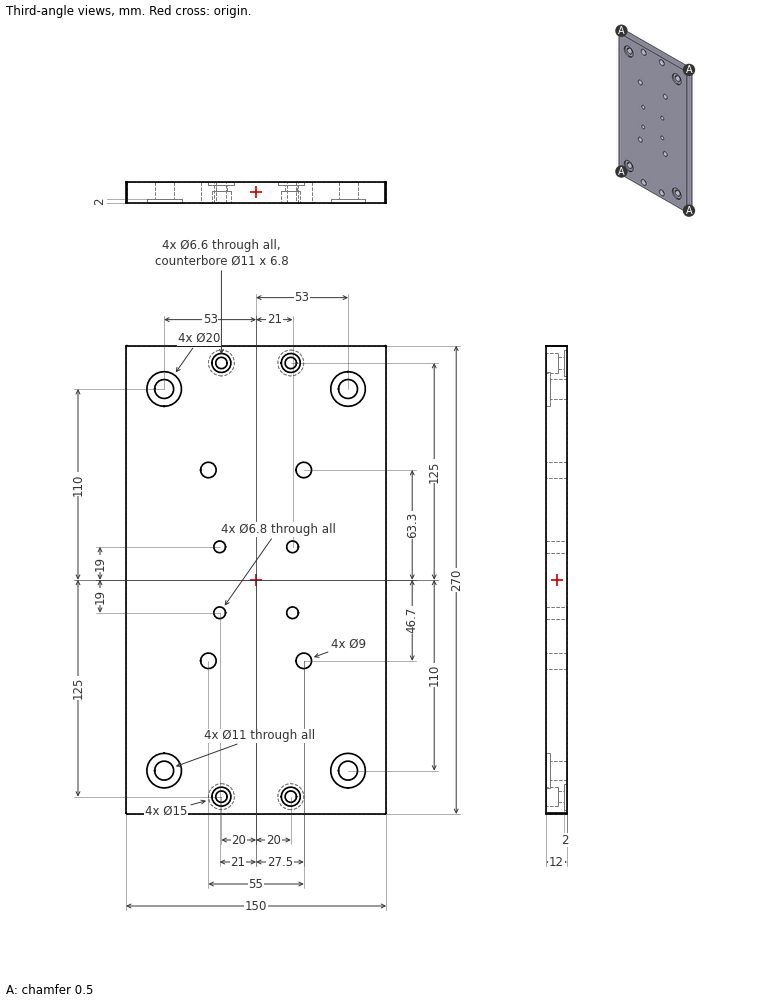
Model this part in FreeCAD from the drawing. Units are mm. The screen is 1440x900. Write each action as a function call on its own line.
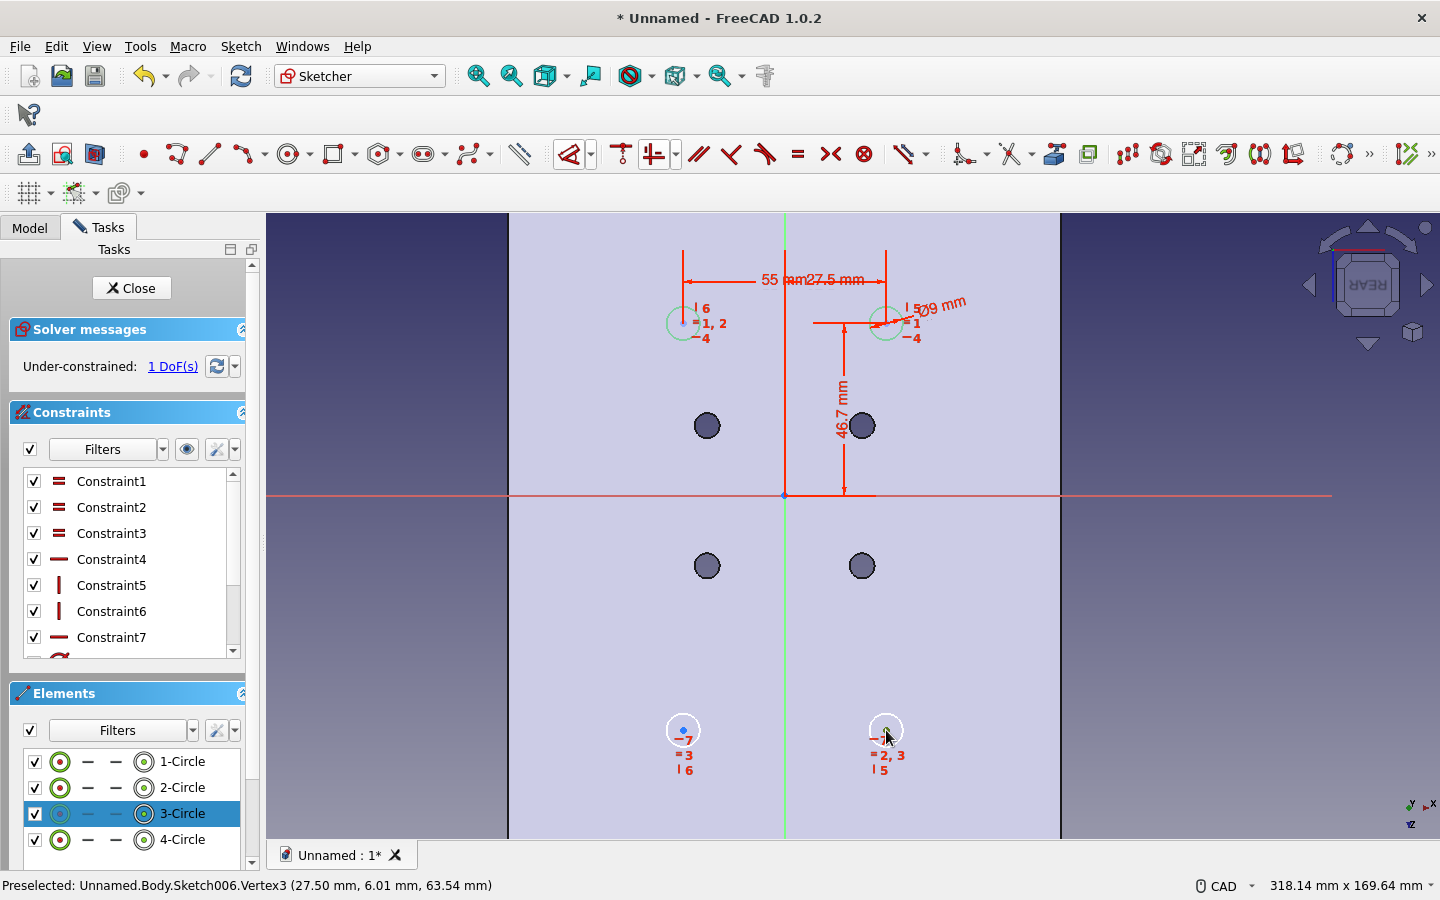
key(i)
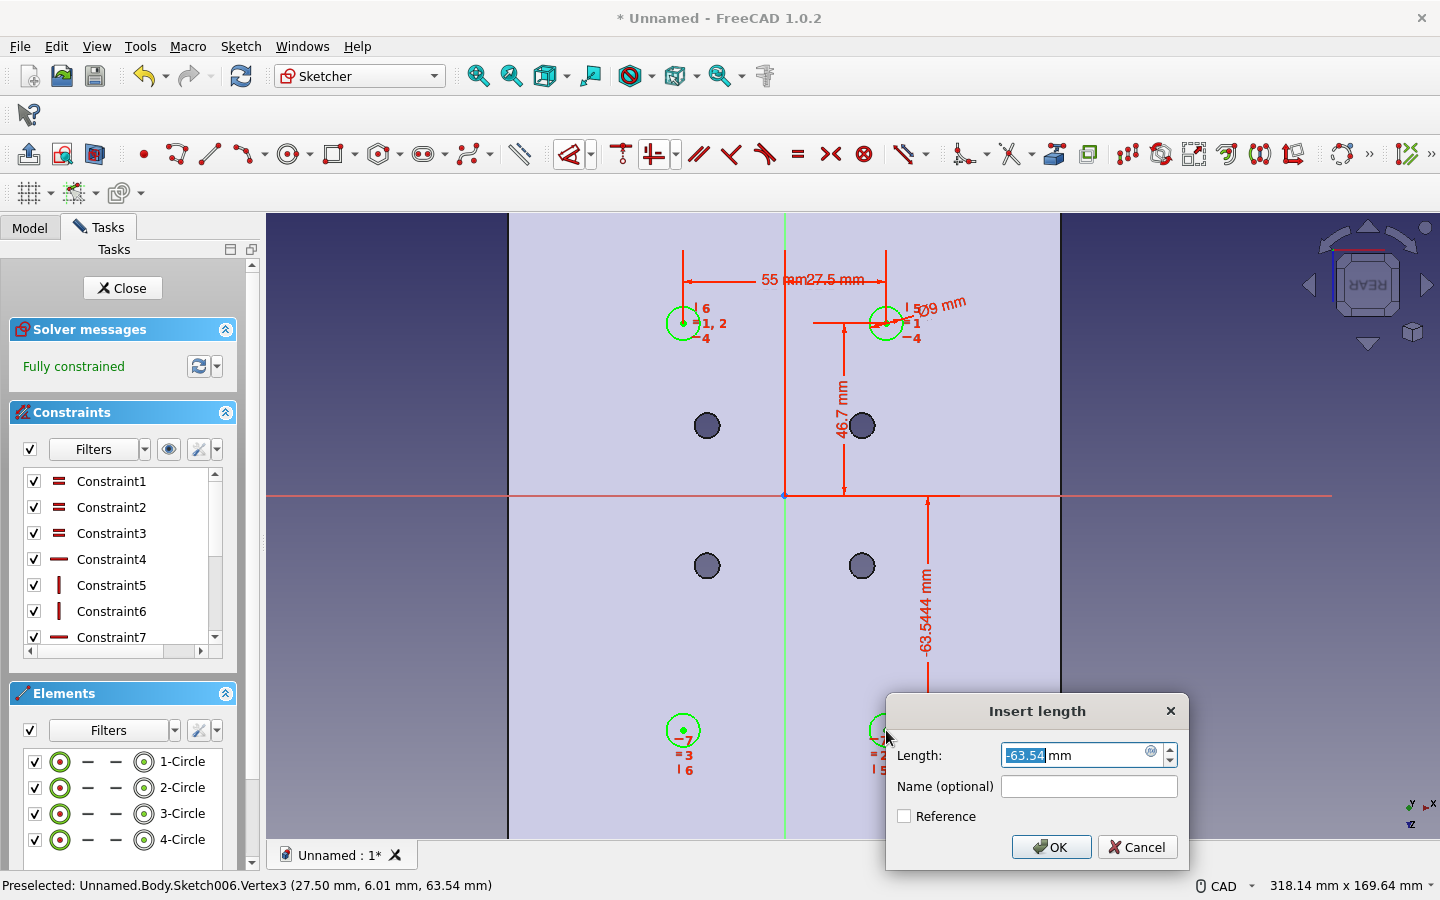
text(-63.3)
key(Return)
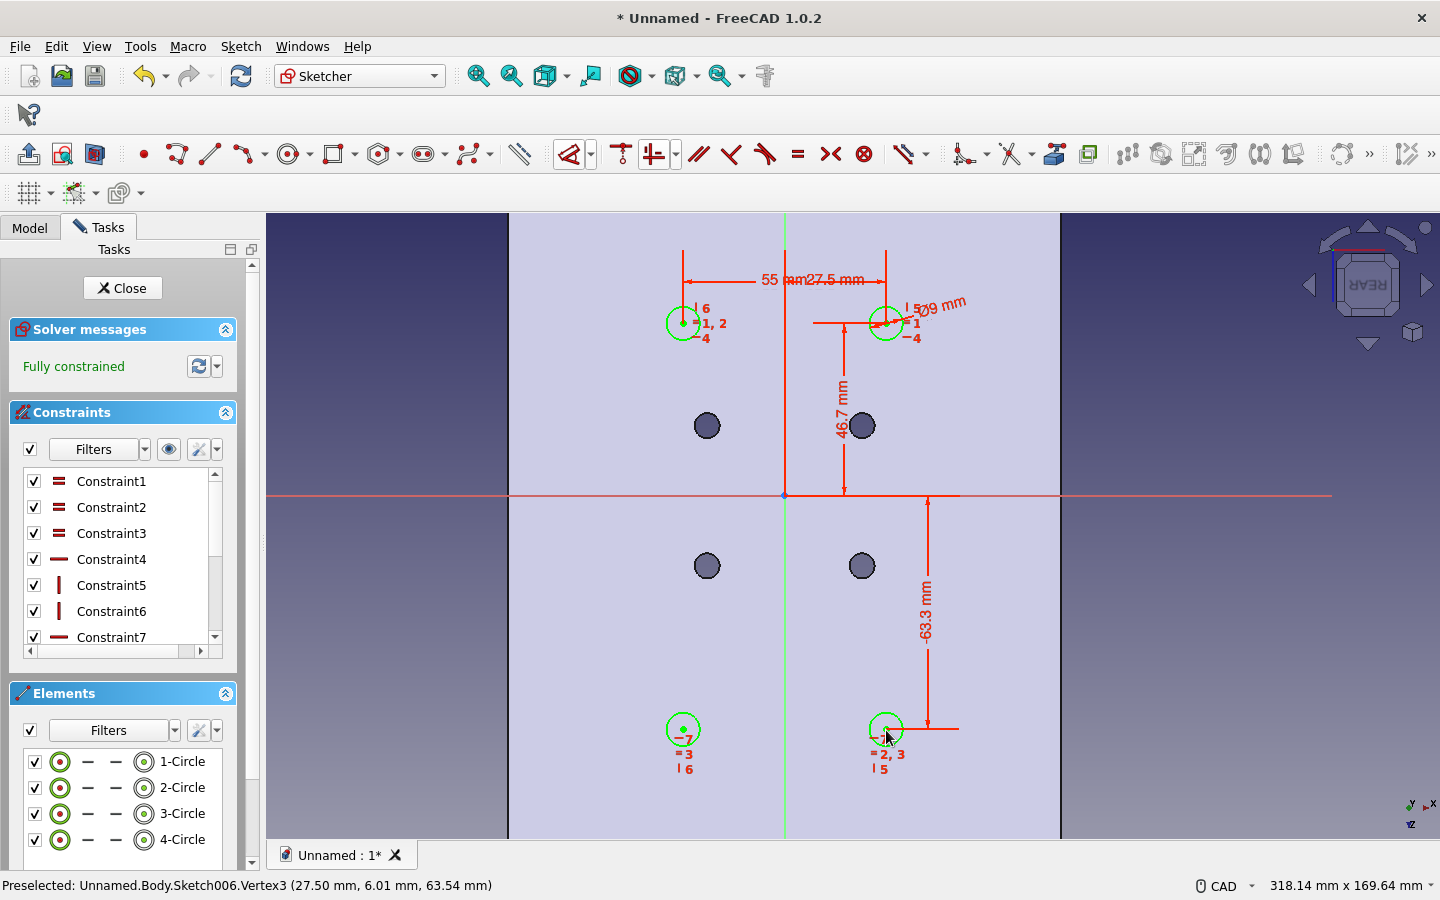
click(123, 288)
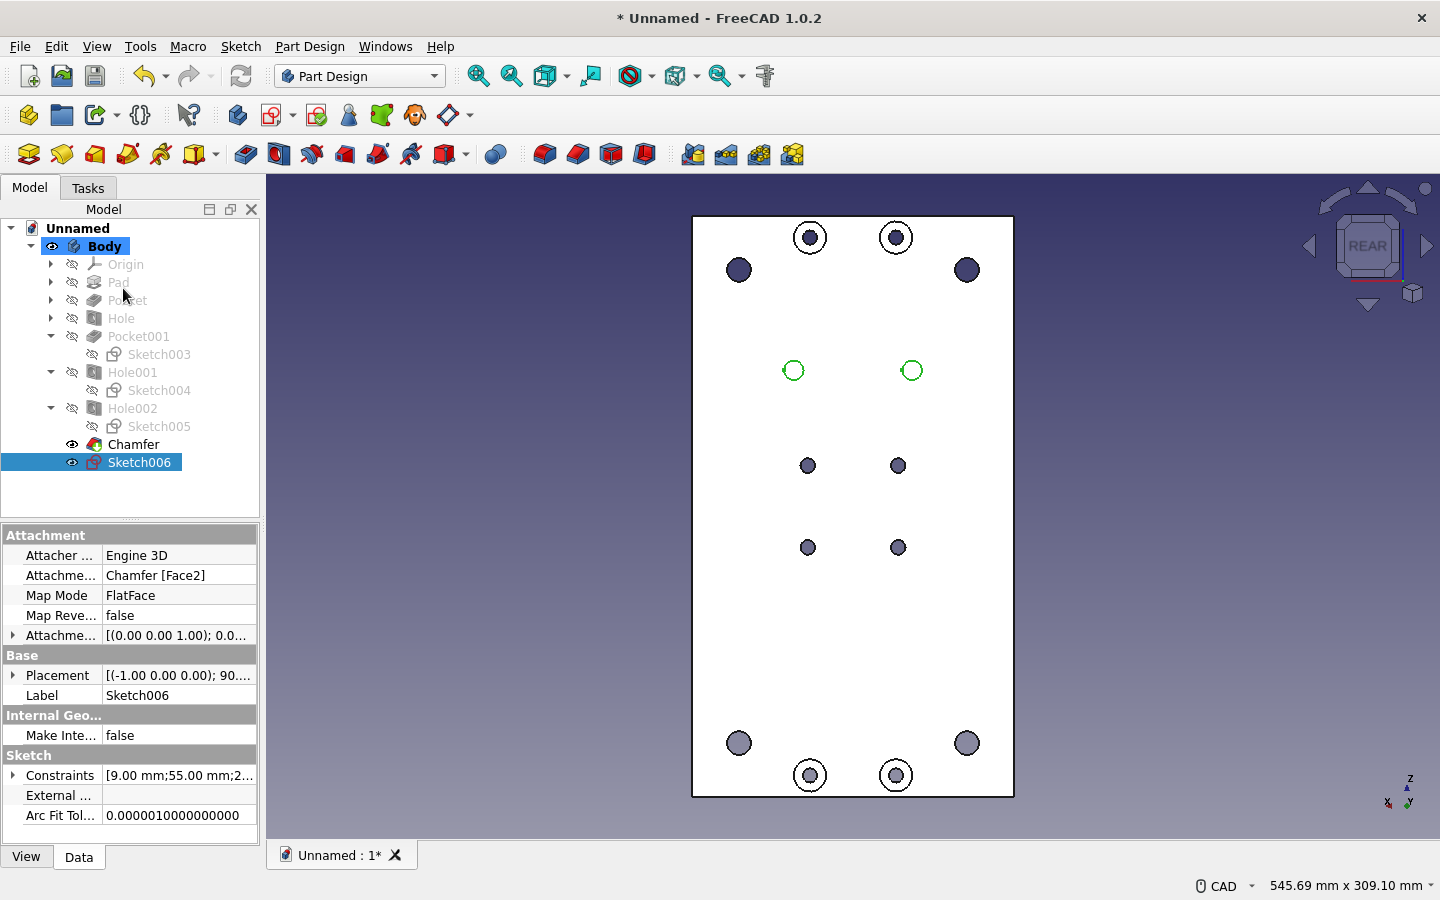
click(246, 154)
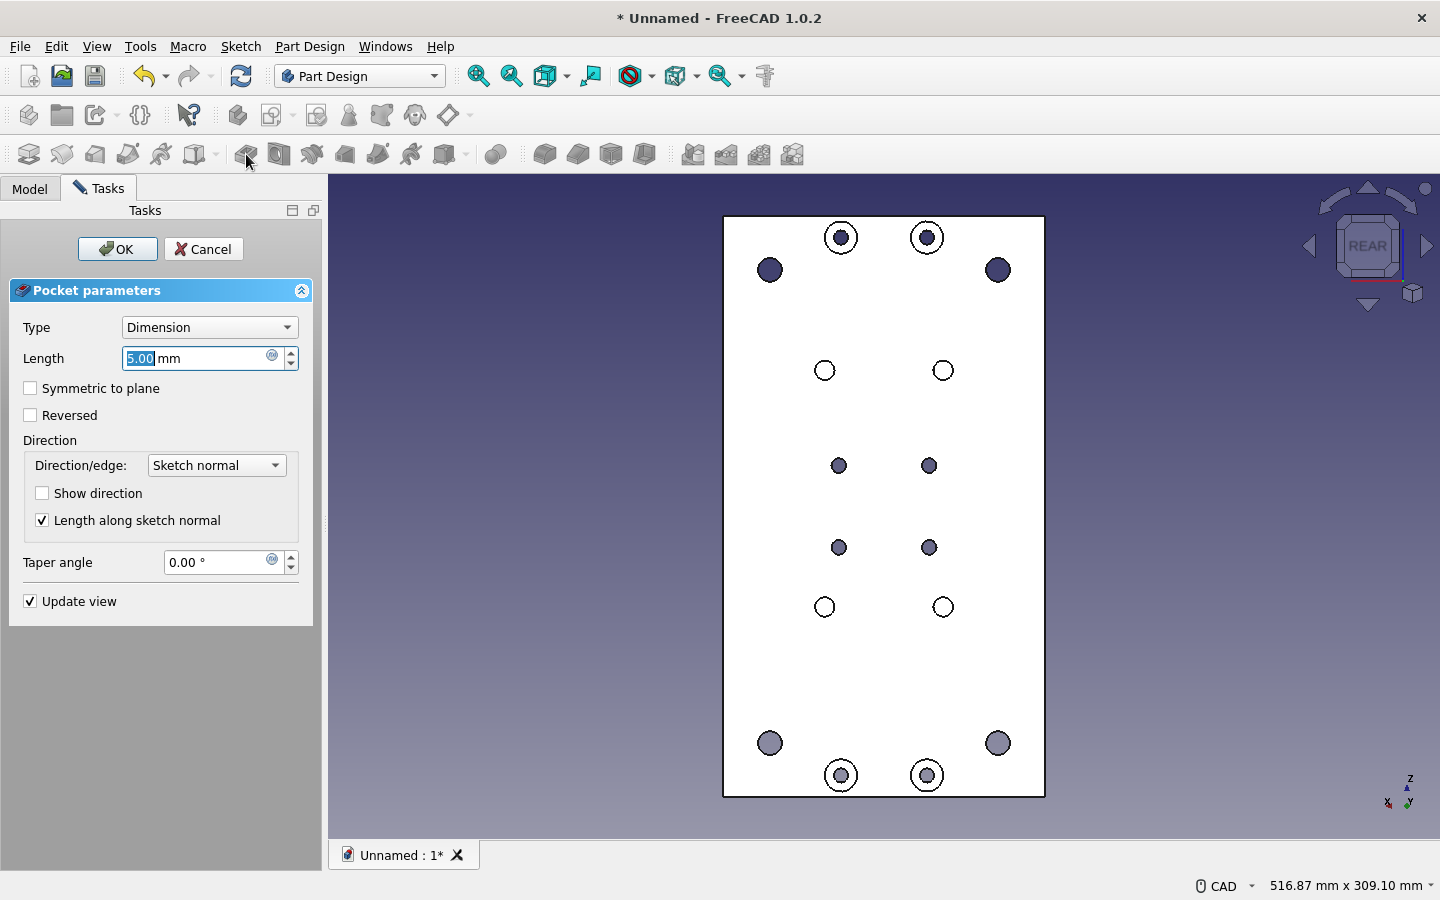
click(210, 328)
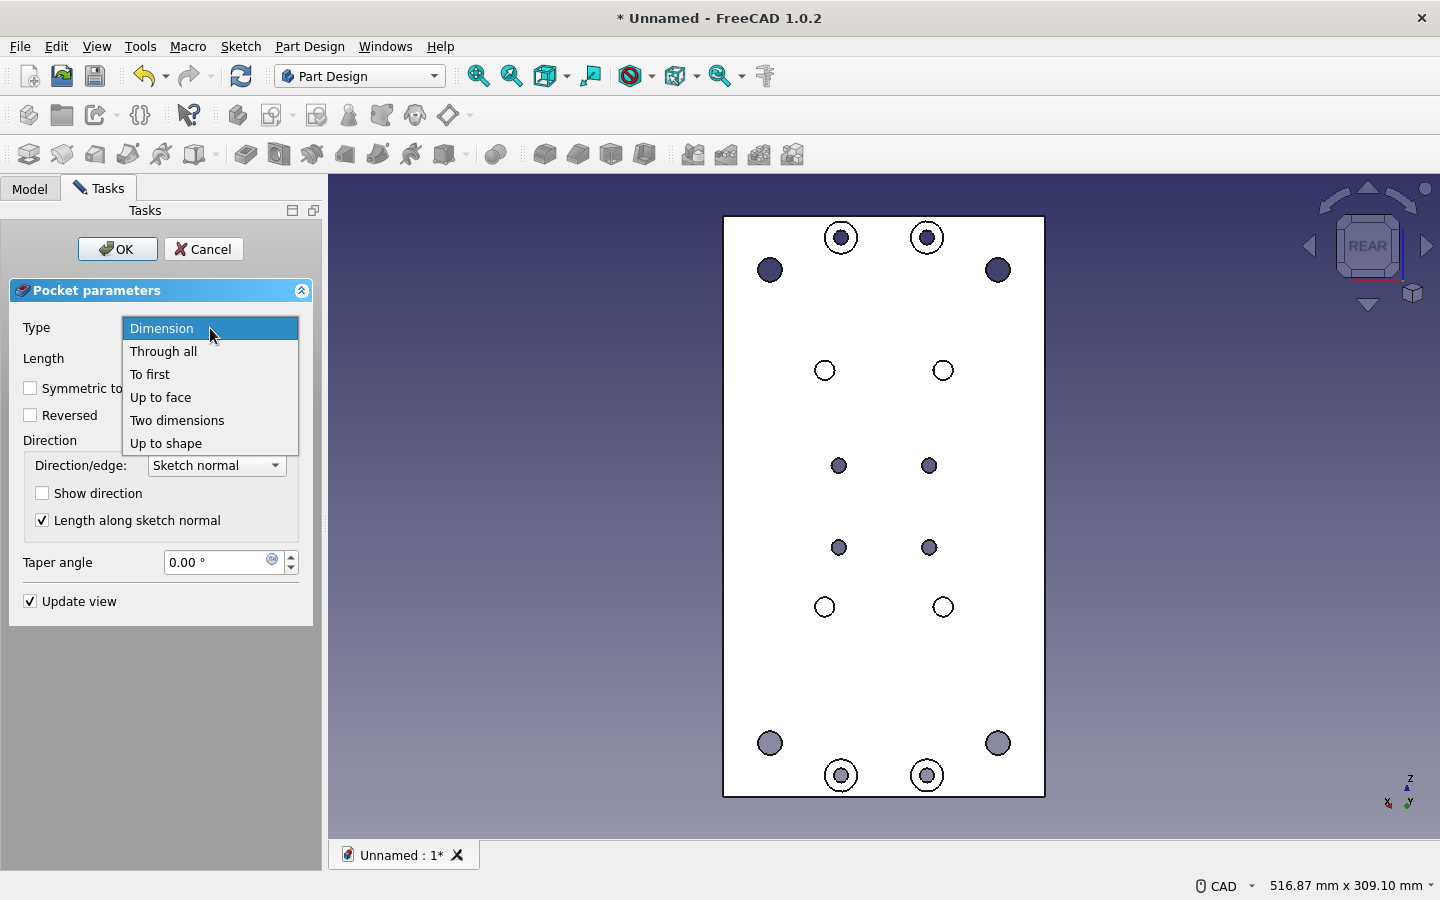
click(208, 352)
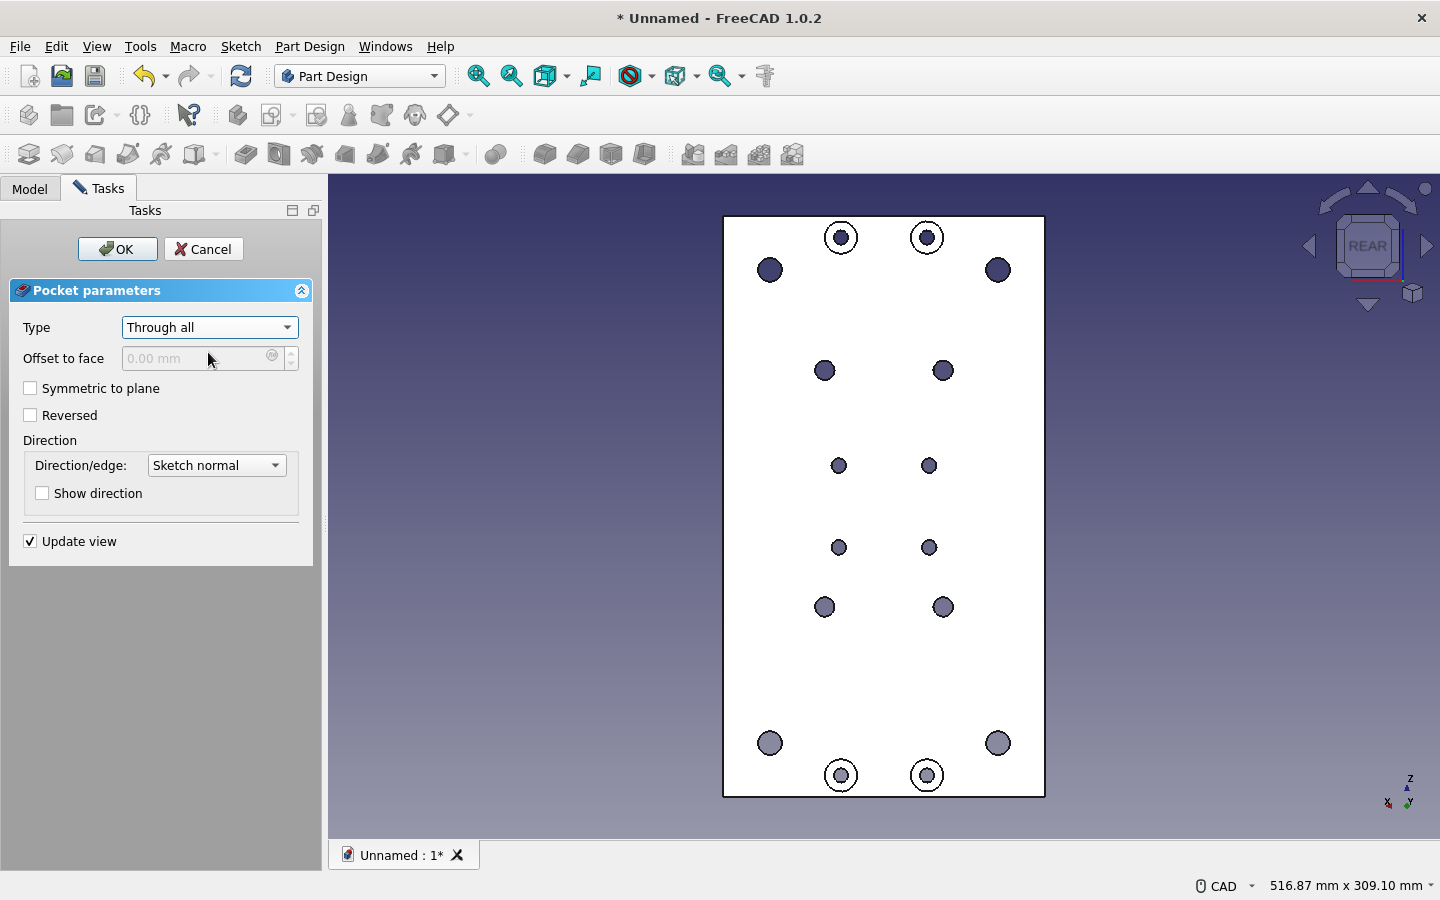
click(118, 249)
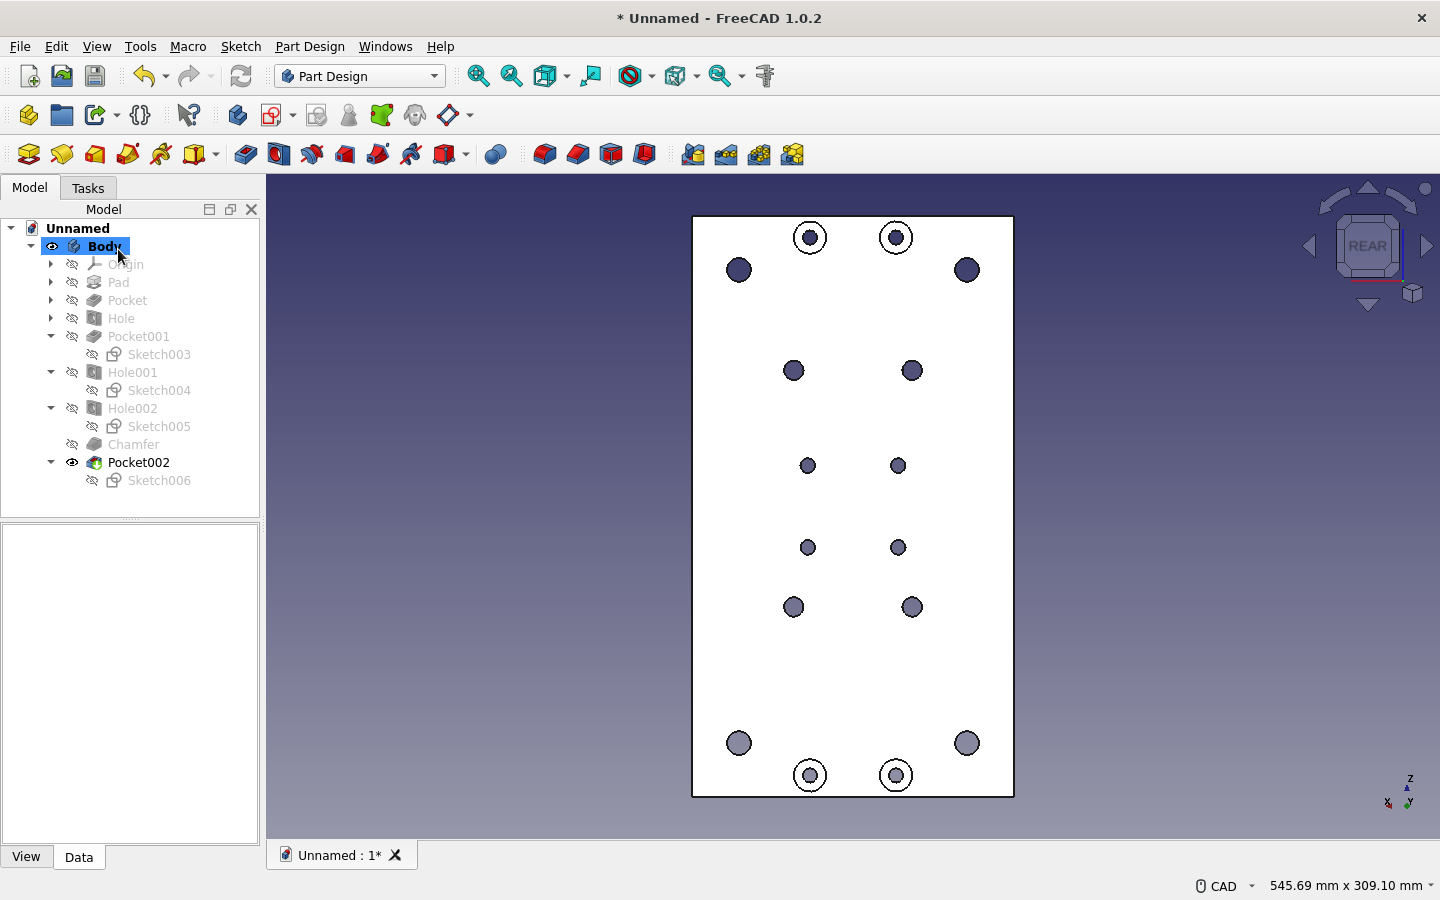
key(0)